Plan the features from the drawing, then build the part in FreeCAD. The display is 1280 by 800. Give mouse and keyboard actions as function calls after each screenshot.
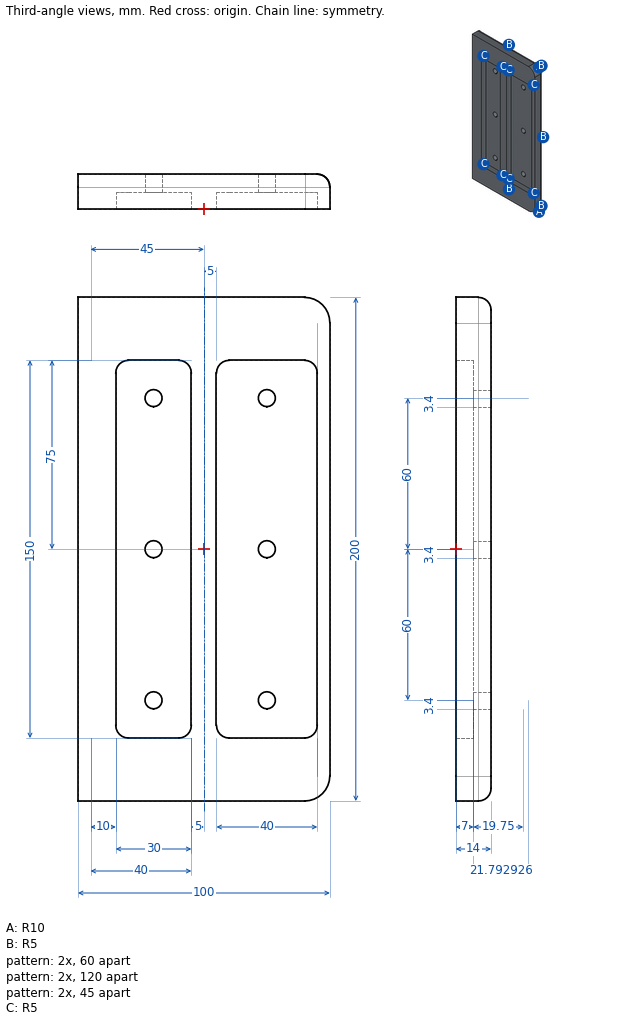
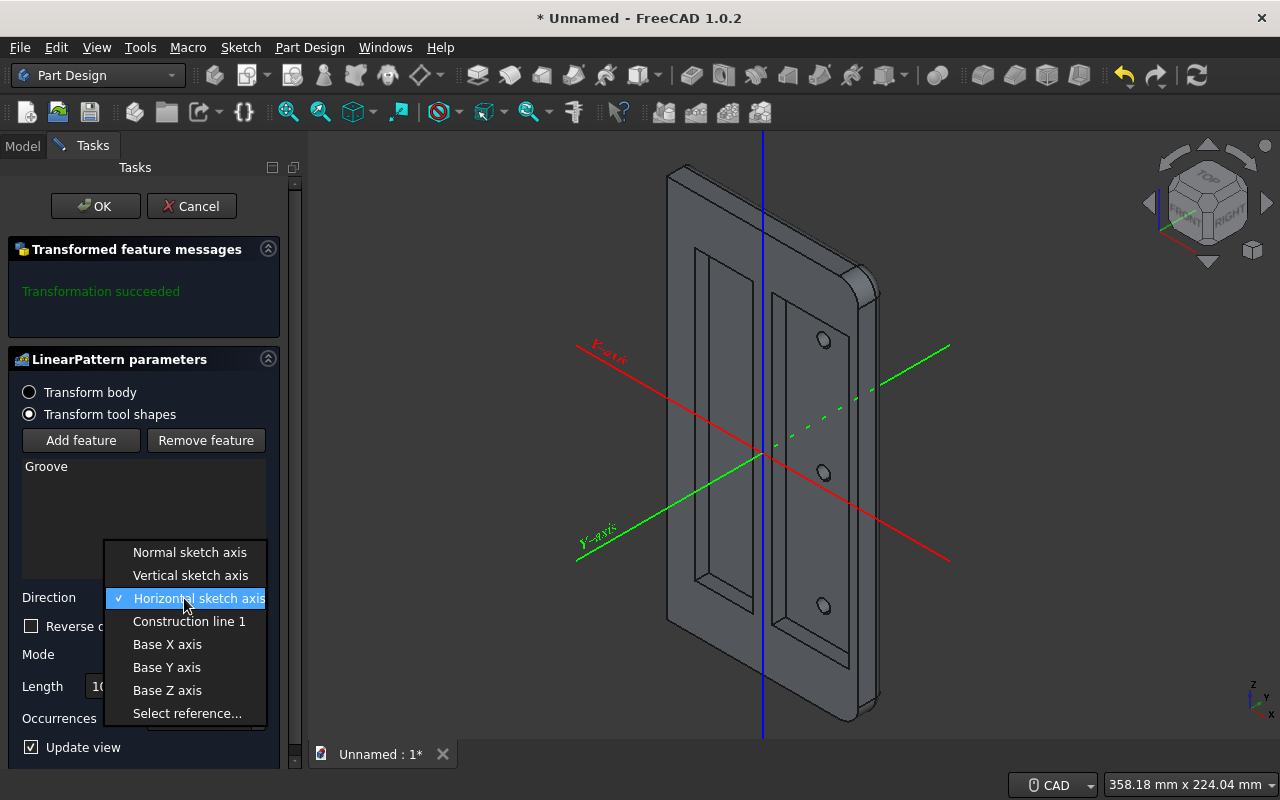
click(184, 644)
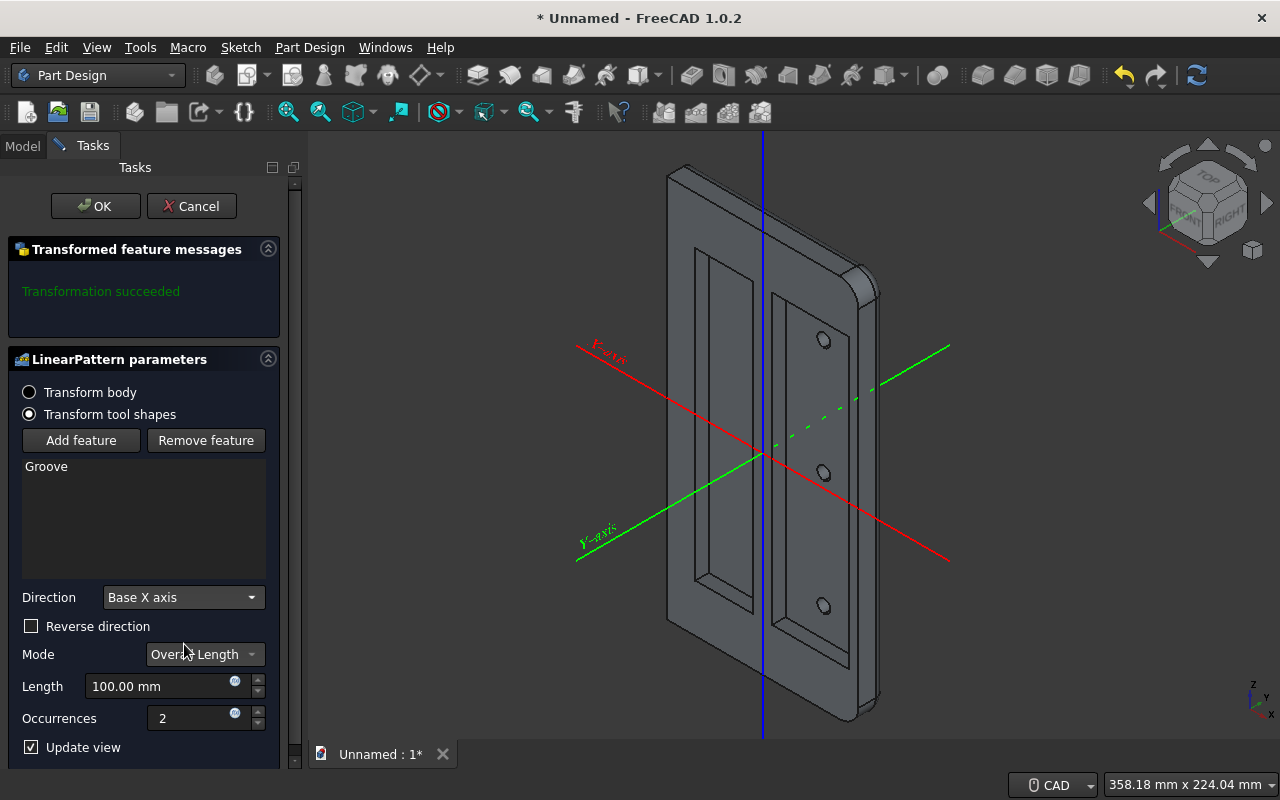
click(206, 654)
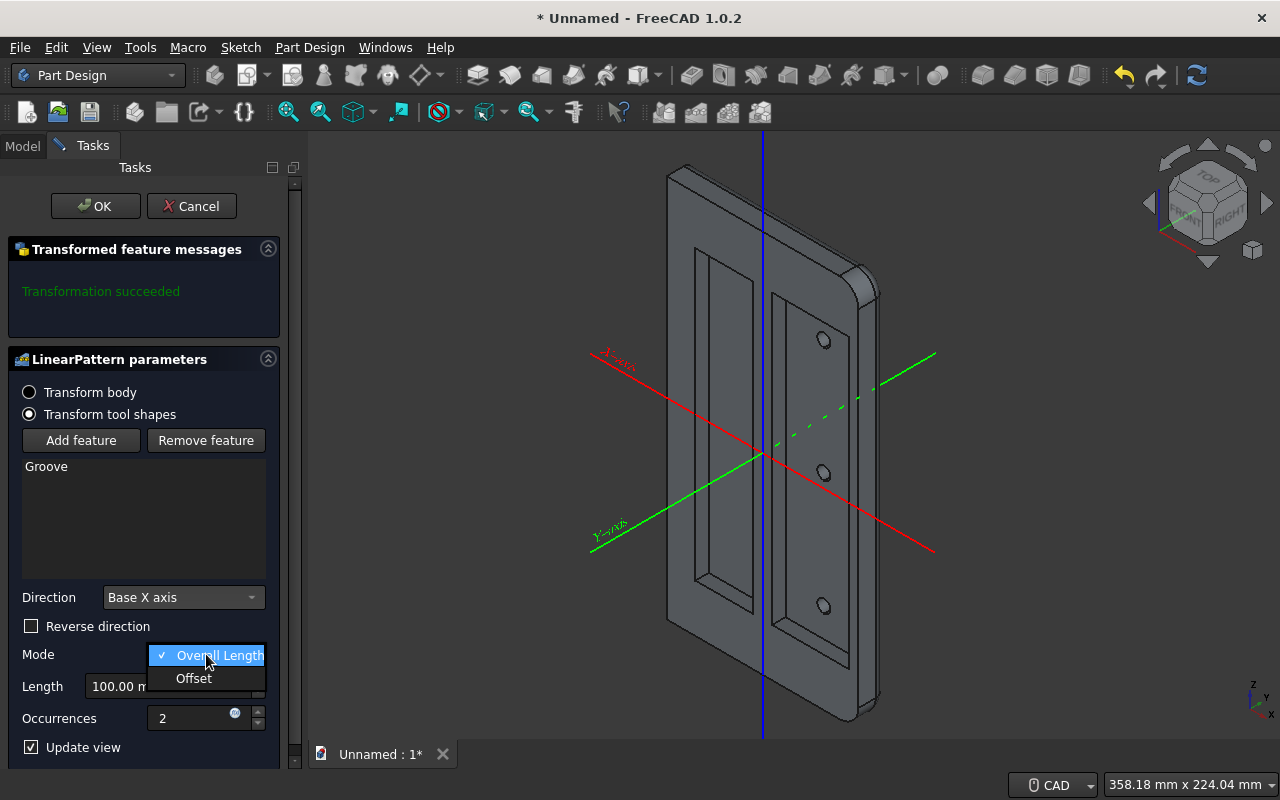
click(206, 678)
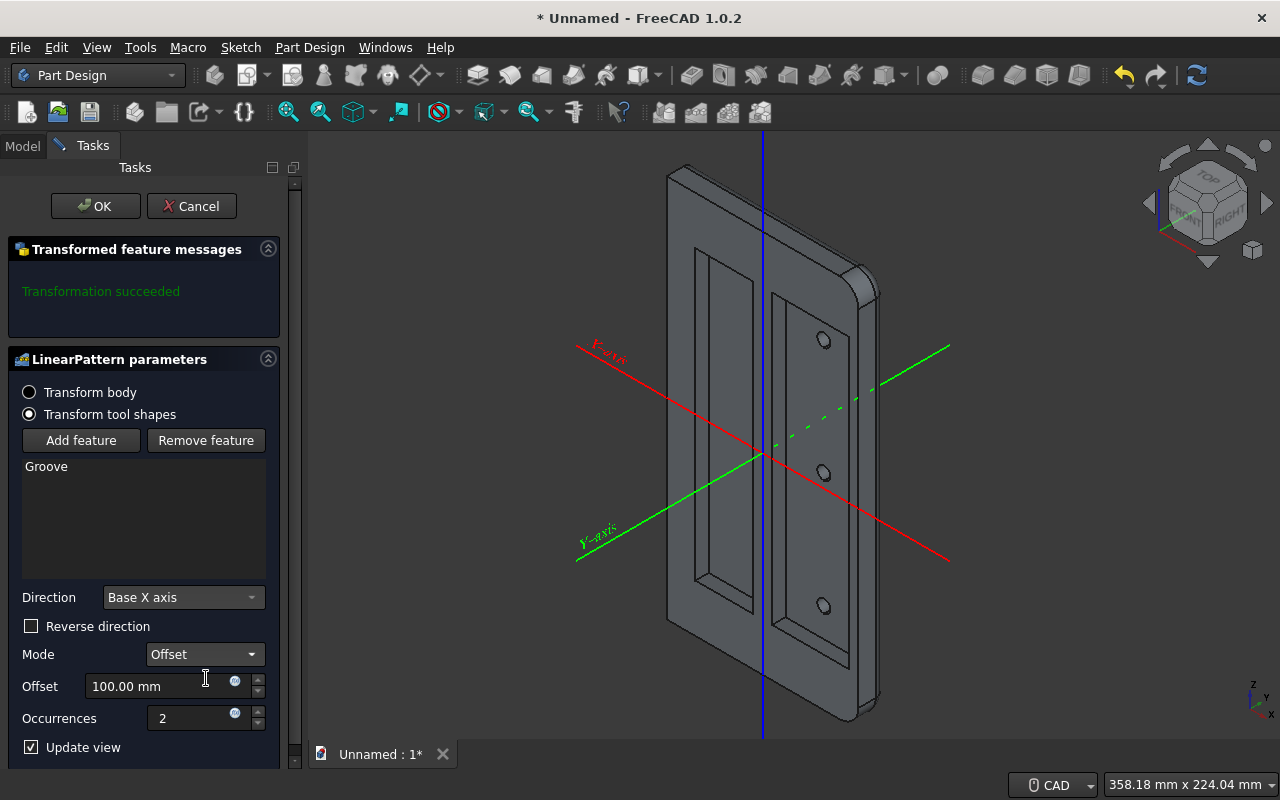
triple_click(168, 686)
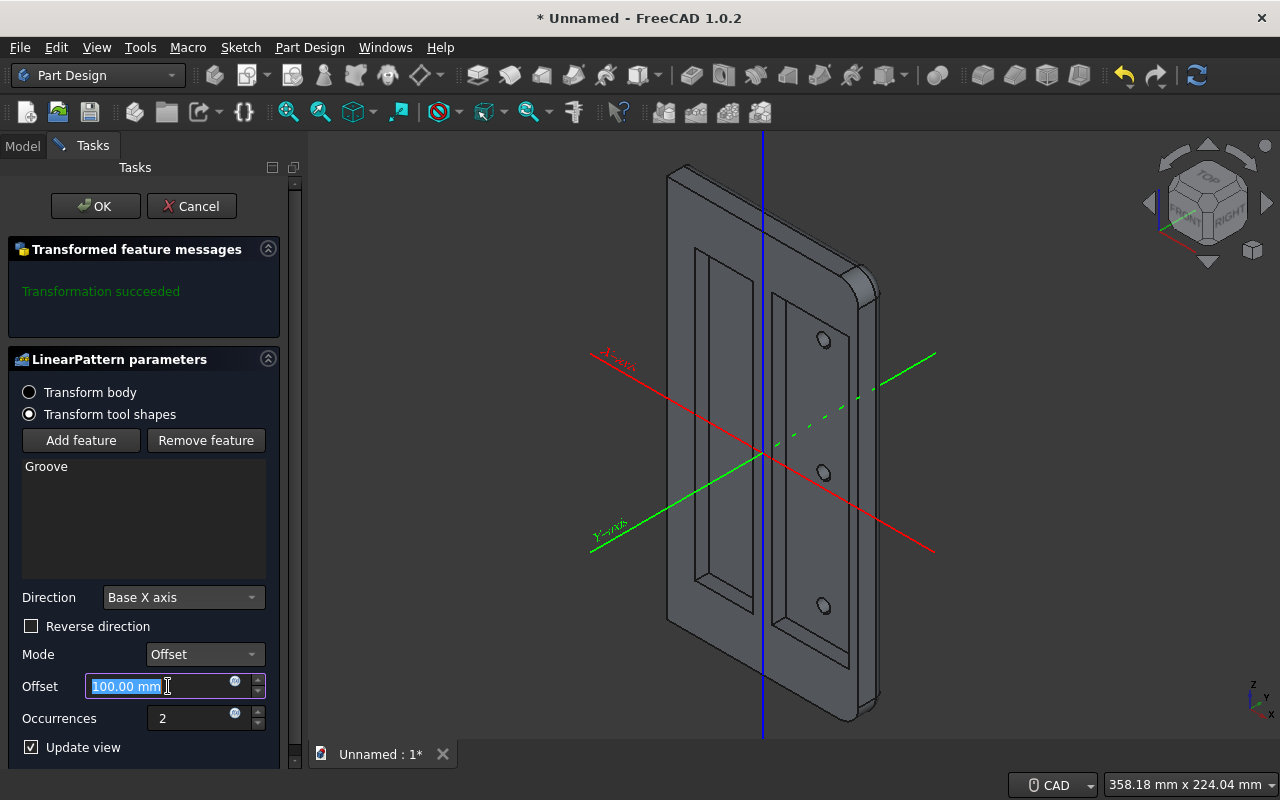
text(45)
key(Tab)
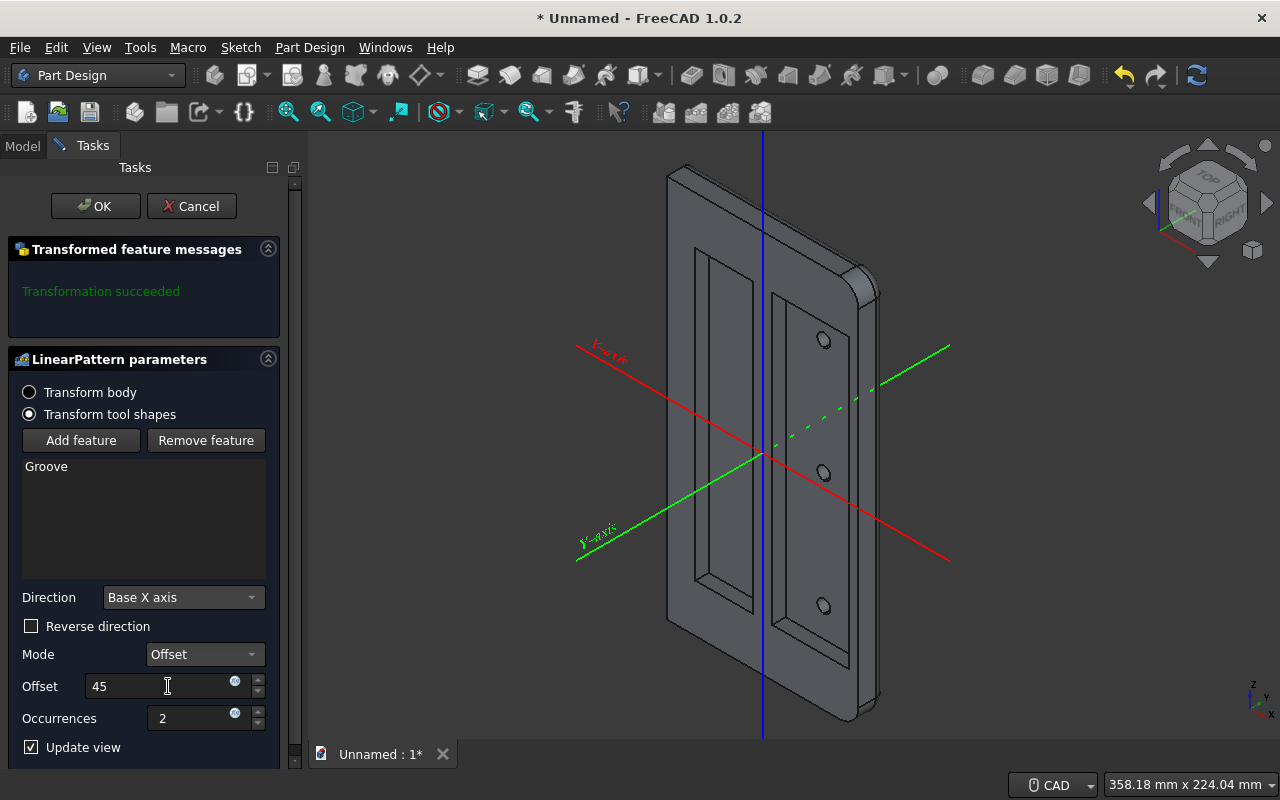
triple_click(198, 718)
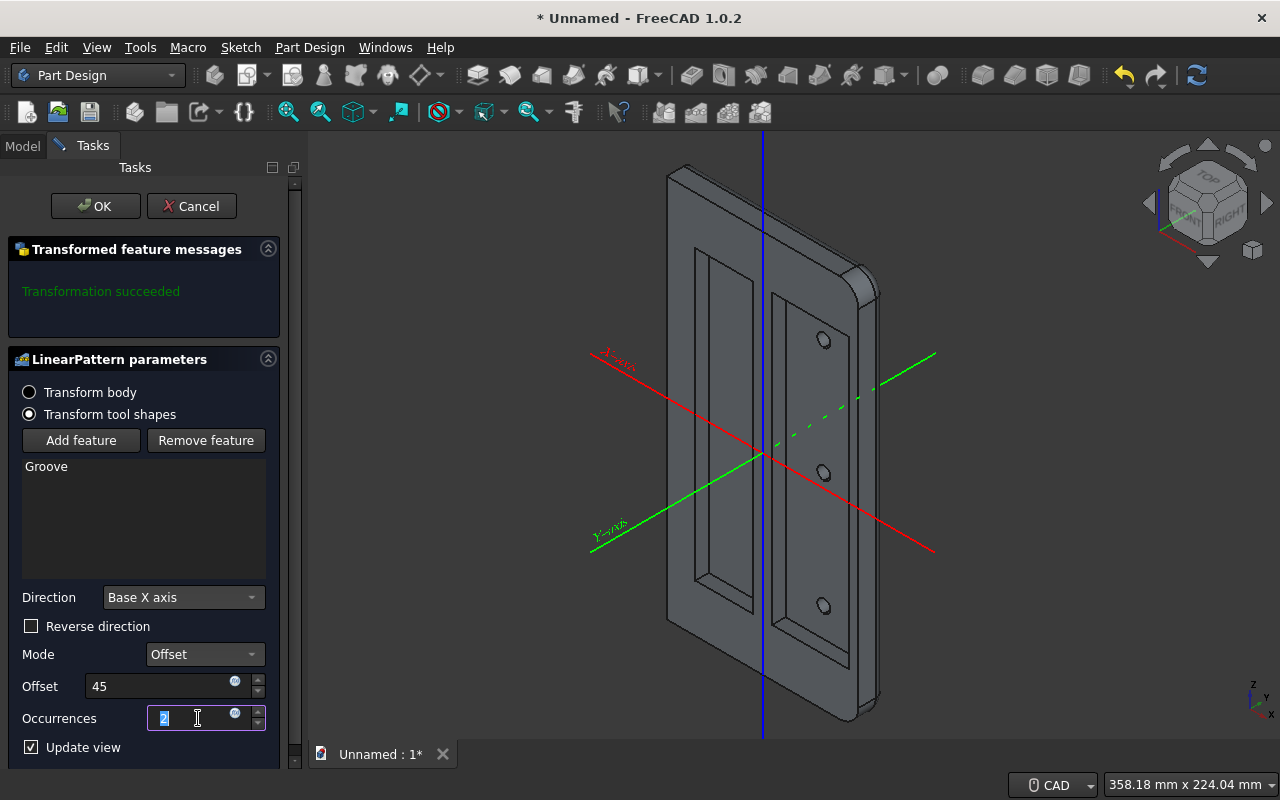
text(2)
key(Tab)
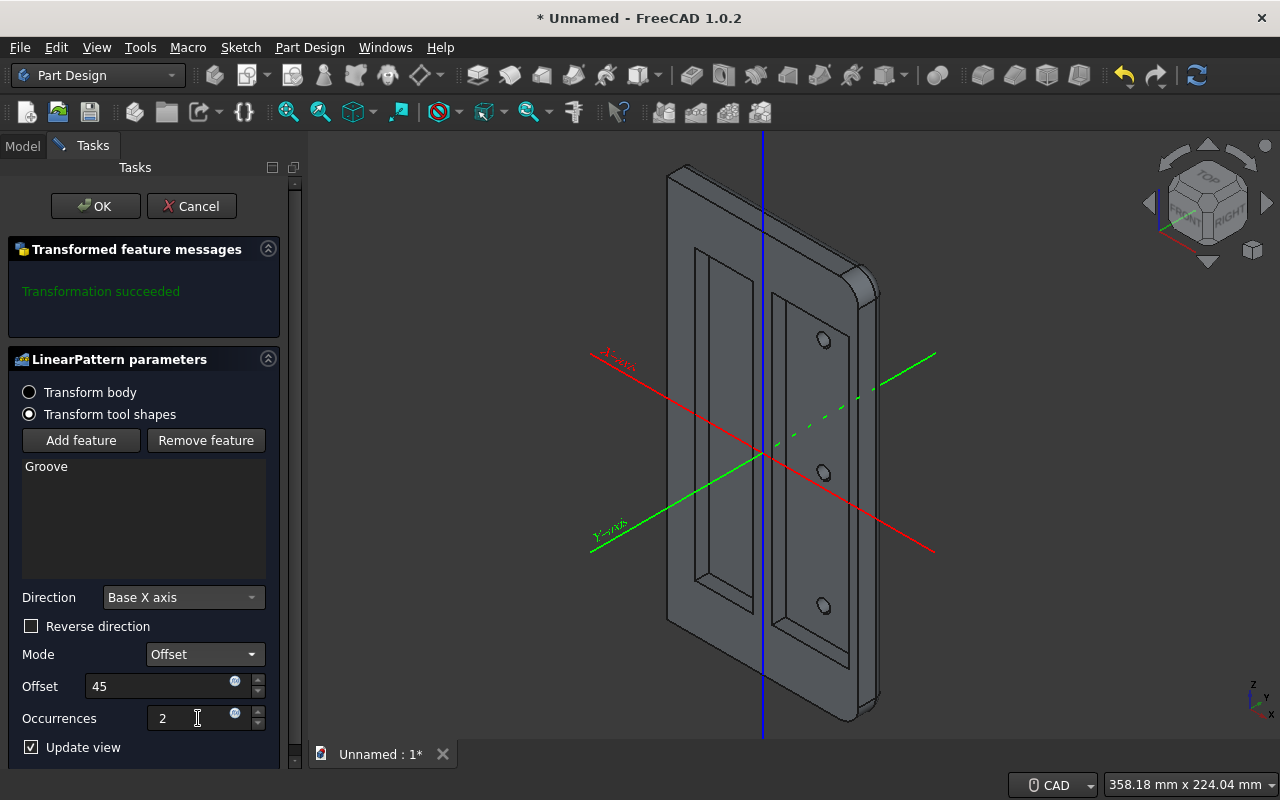
click(30, 626)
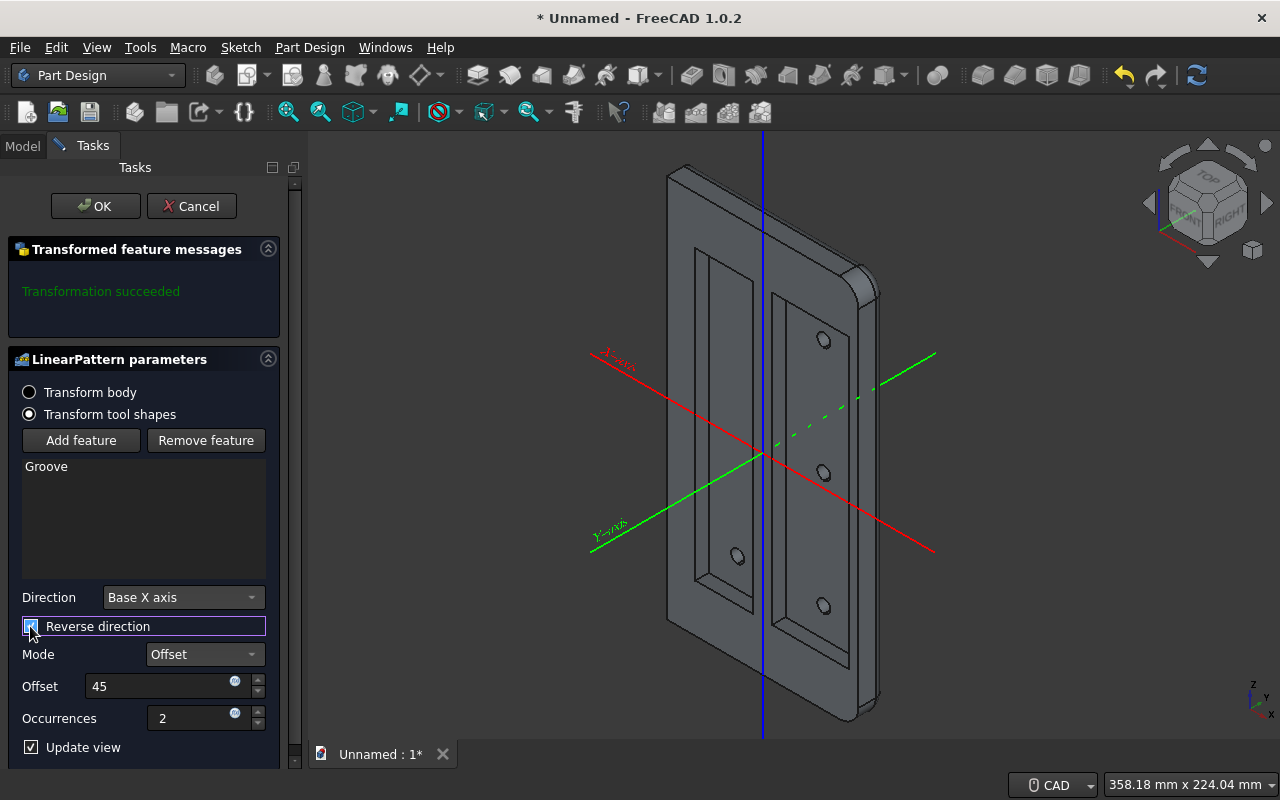
click(96, 206)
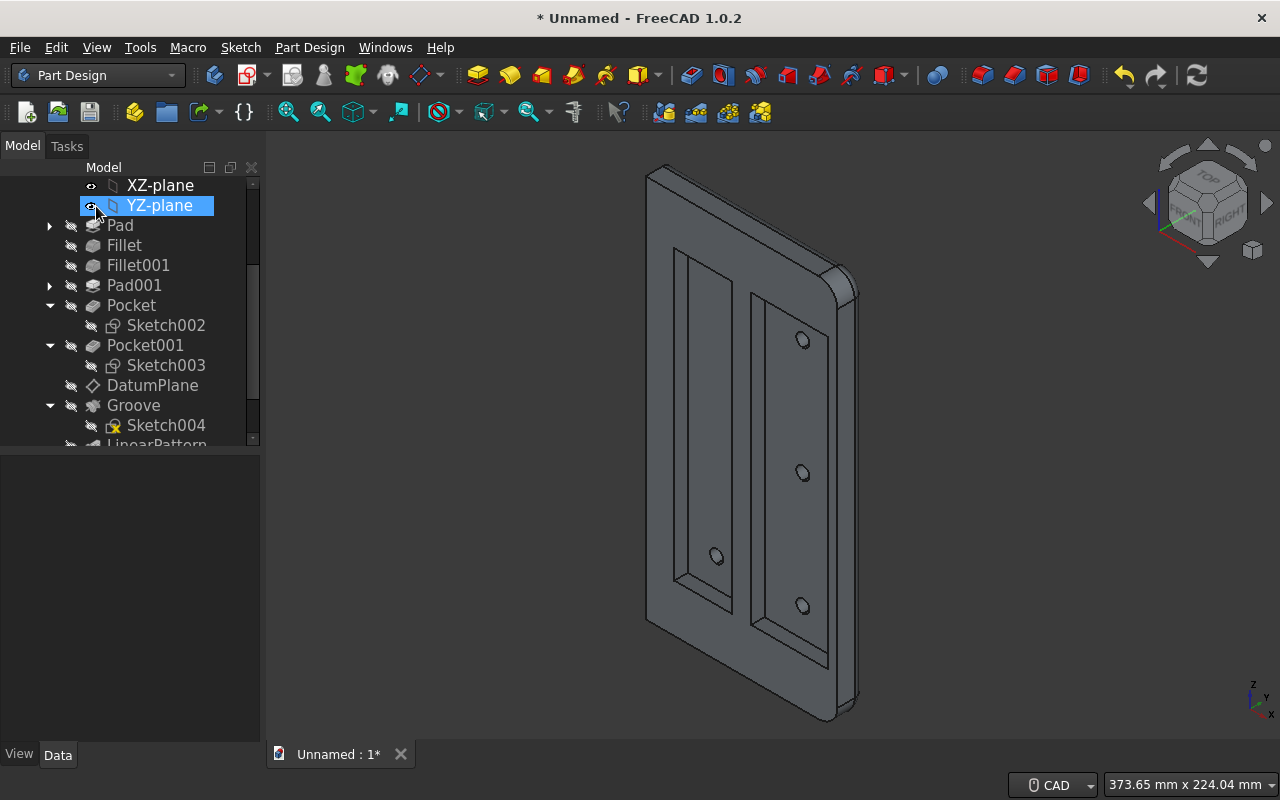
scroll(160, 321, down, 3)